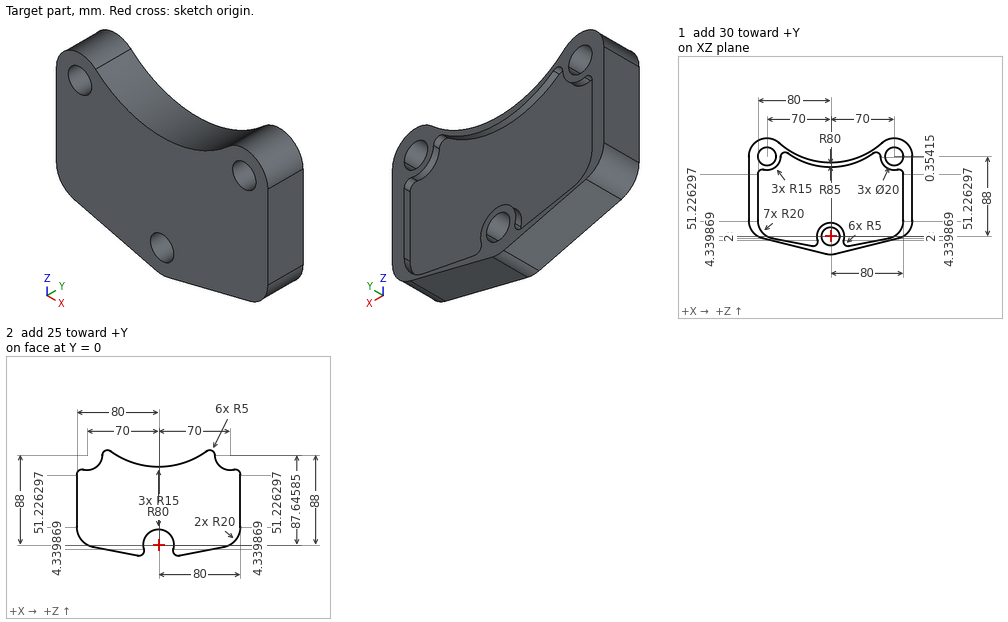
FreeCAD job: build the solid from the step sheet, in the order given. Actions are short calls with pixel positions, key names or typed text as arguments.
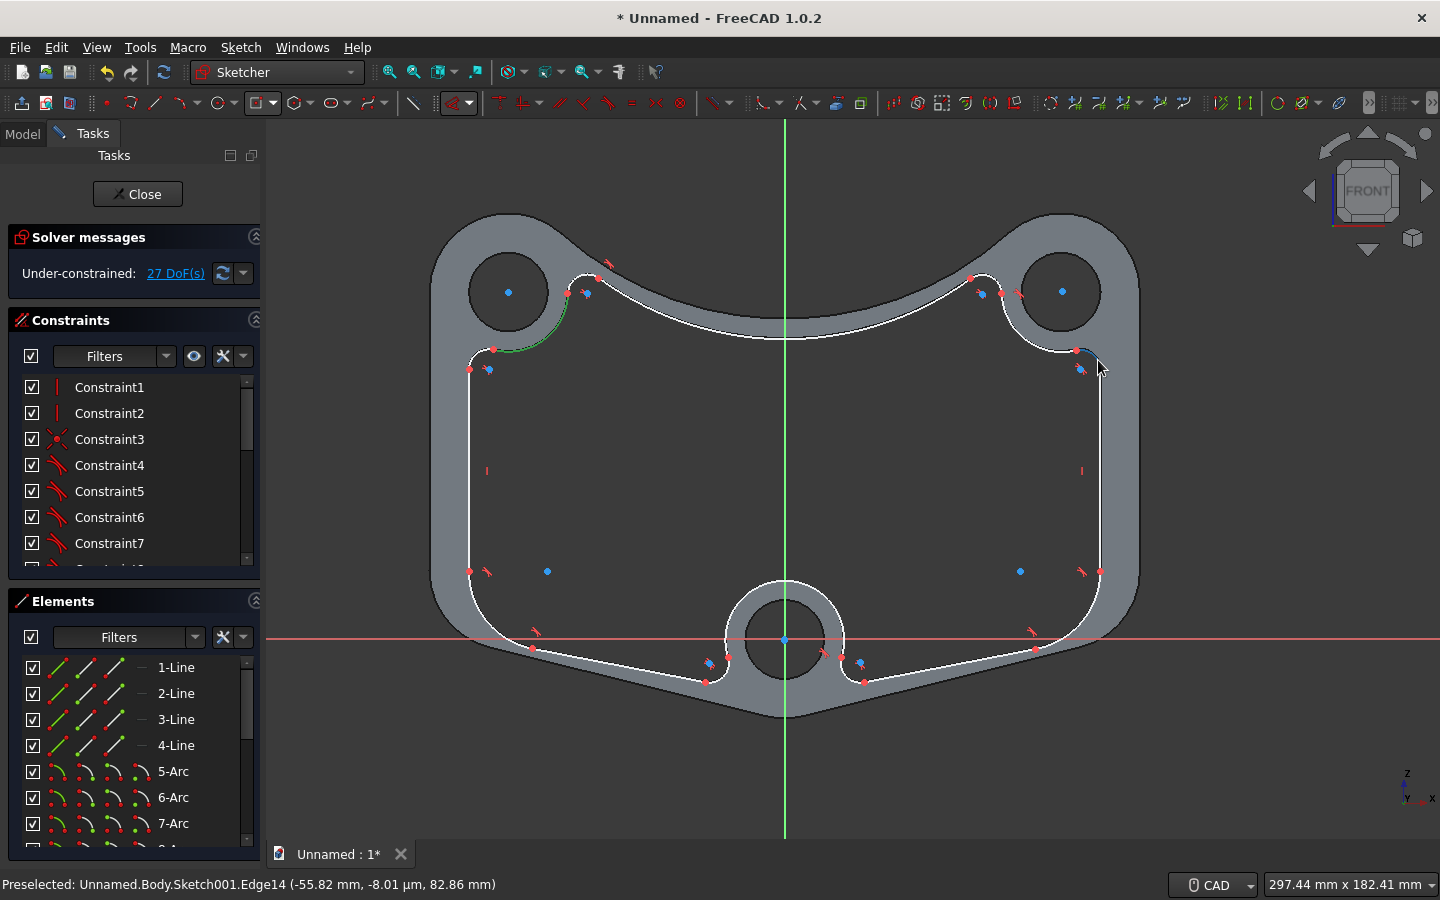
scroll(483, 350, up, 2)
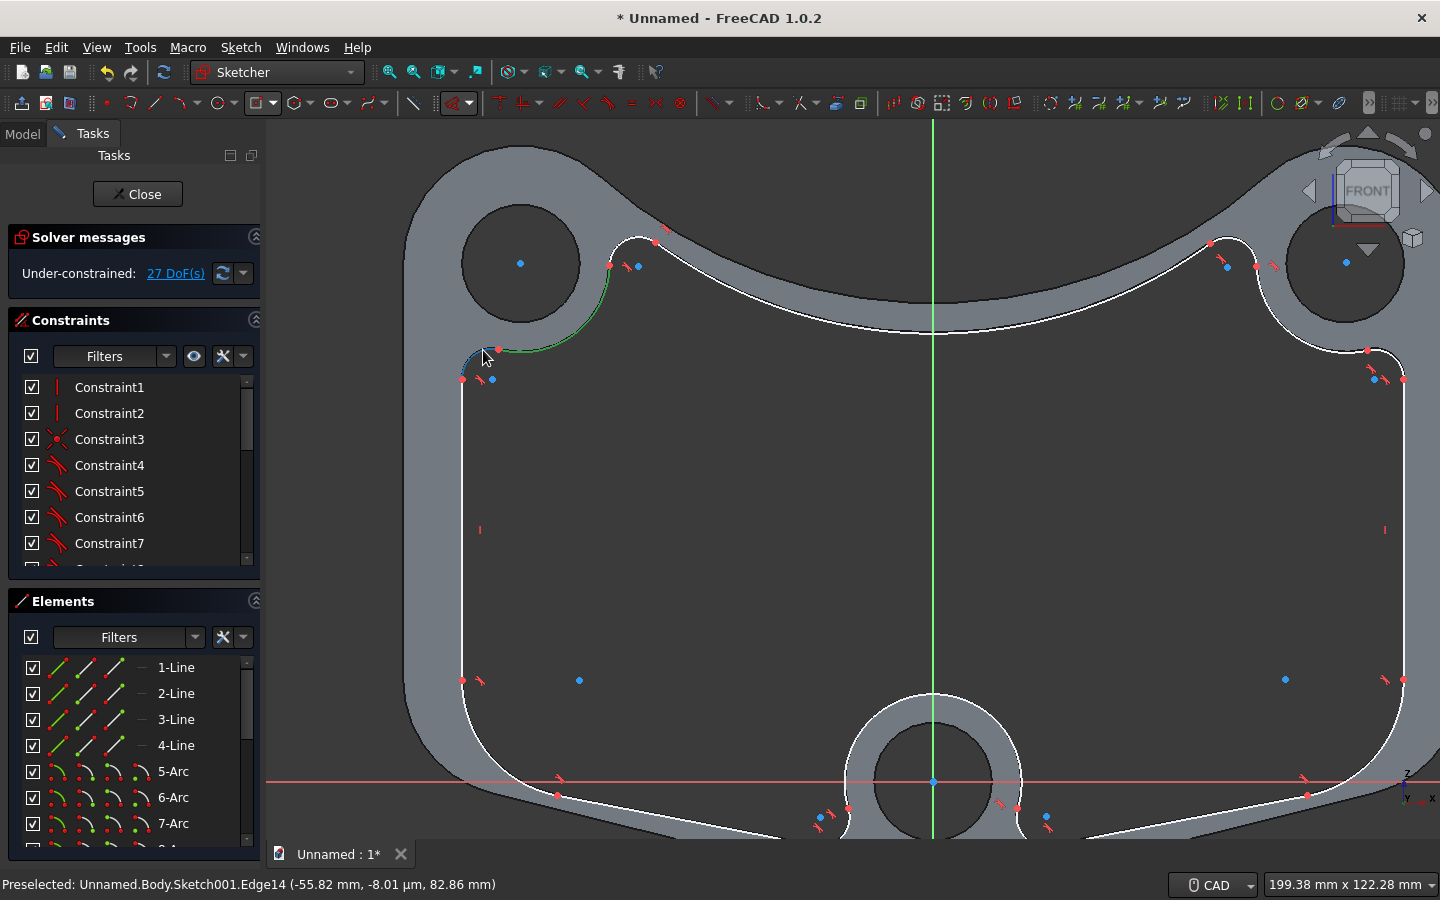
click(483, 350)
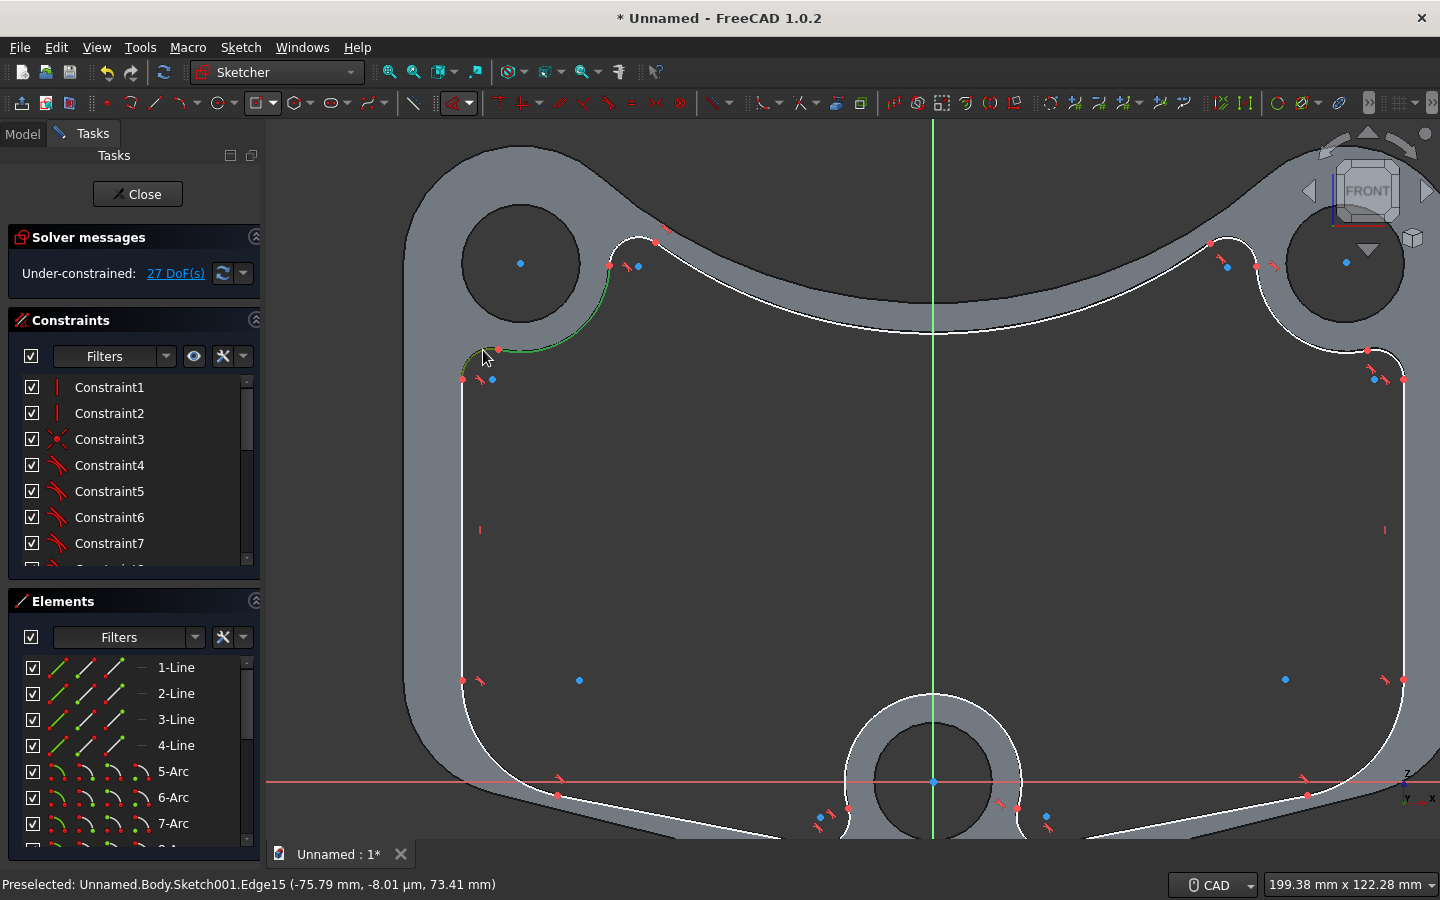
click(608, 104)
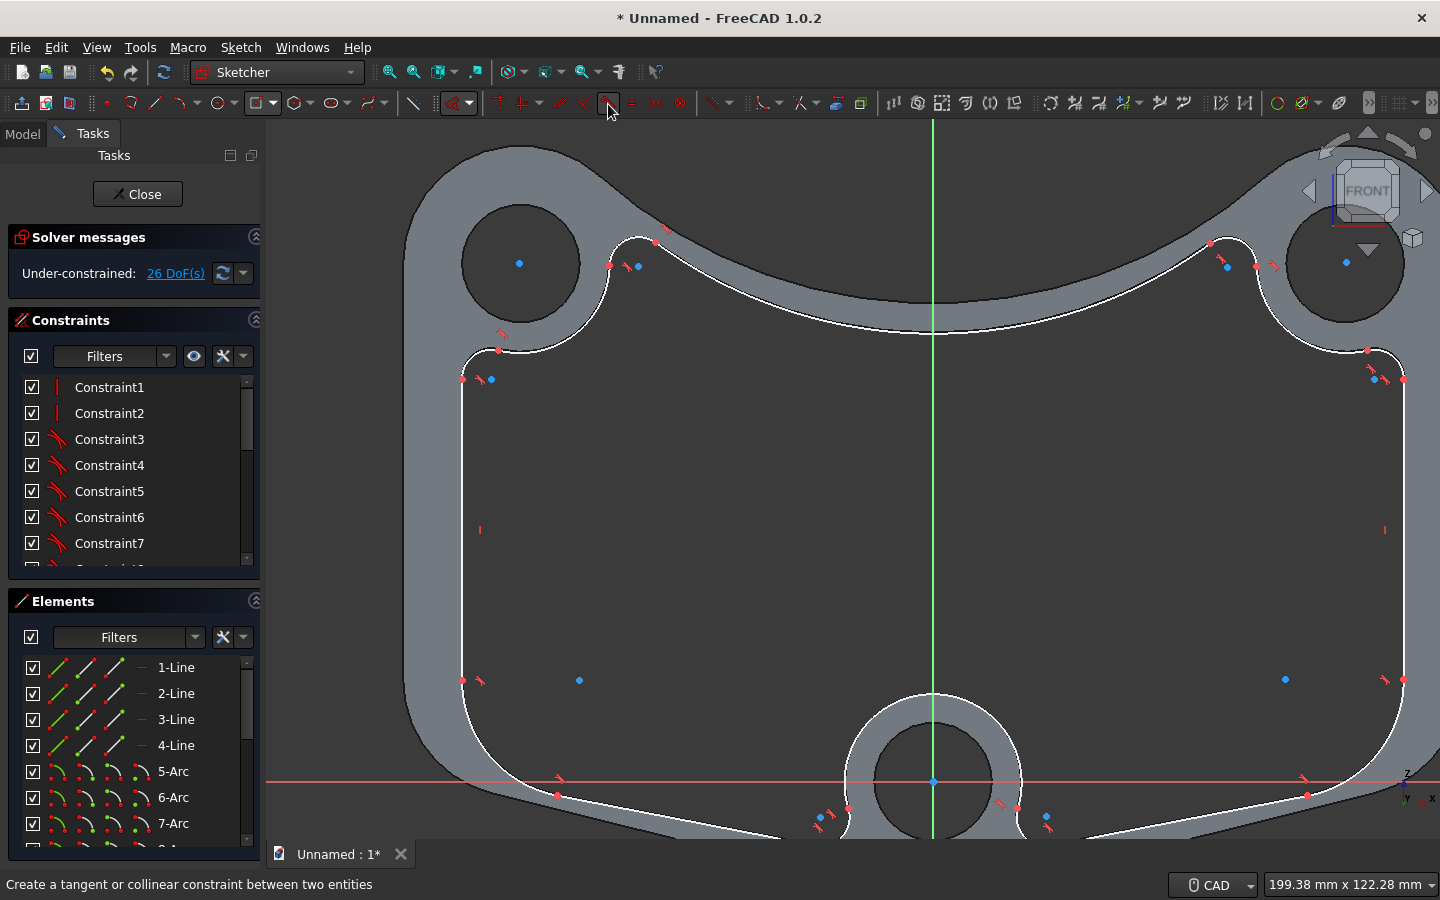
scroll(933, 782, up, 2)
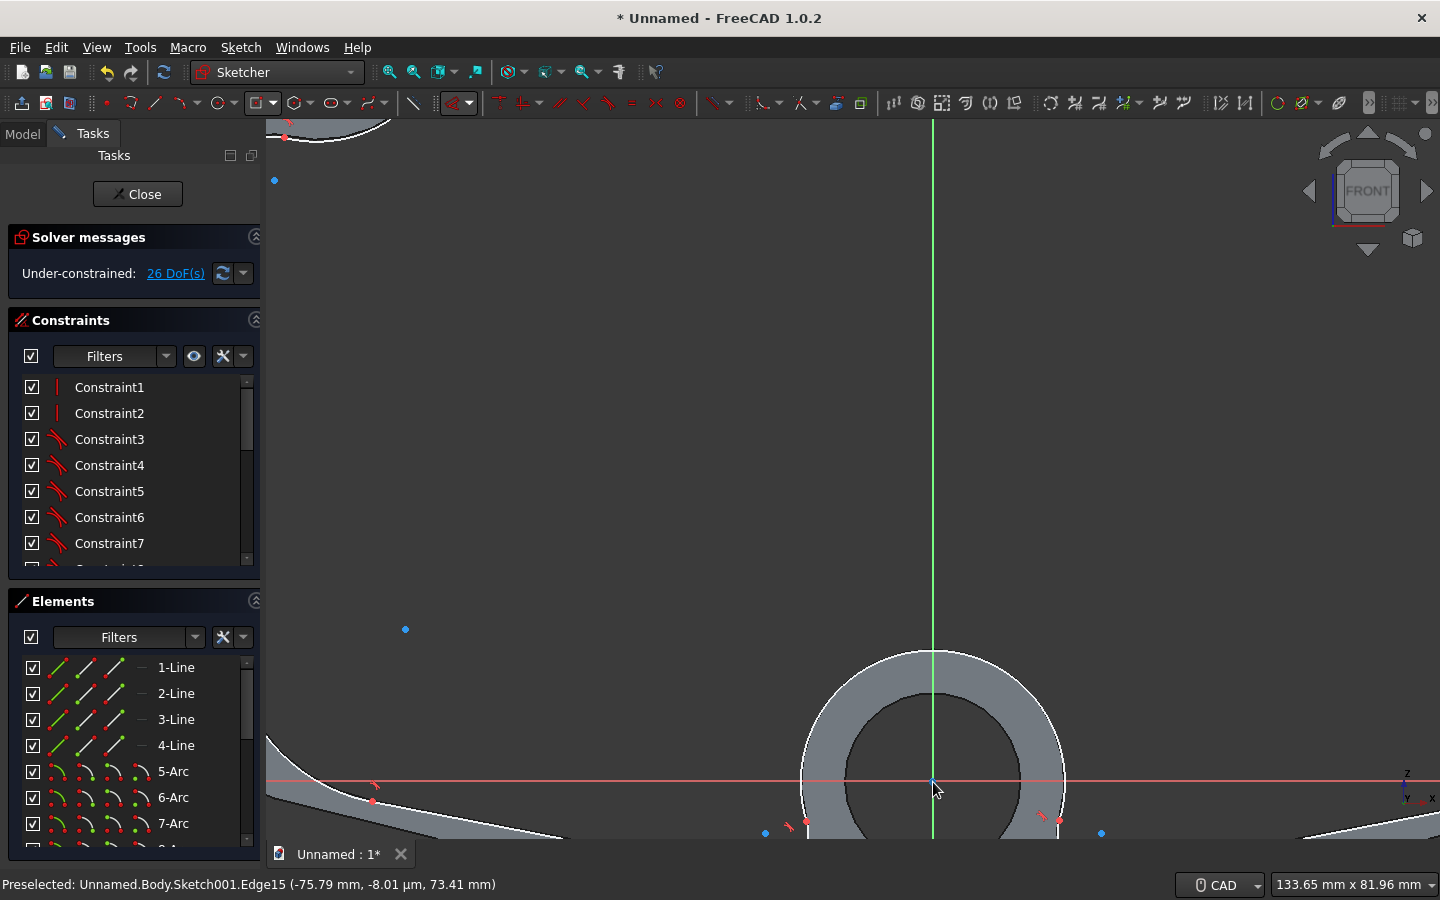
drag(923, 771, 943, 793)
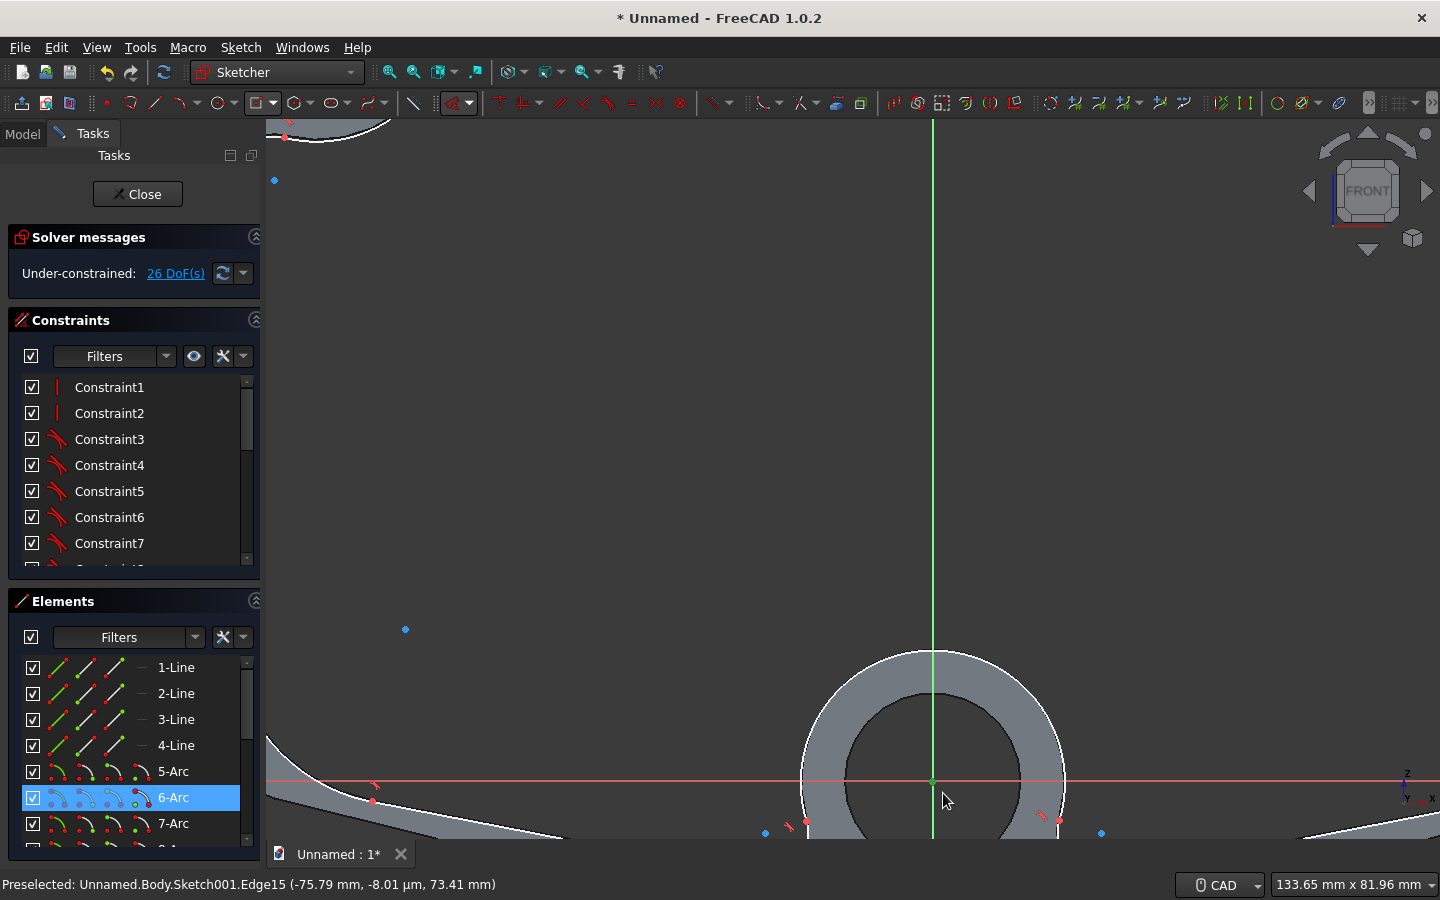
key(c)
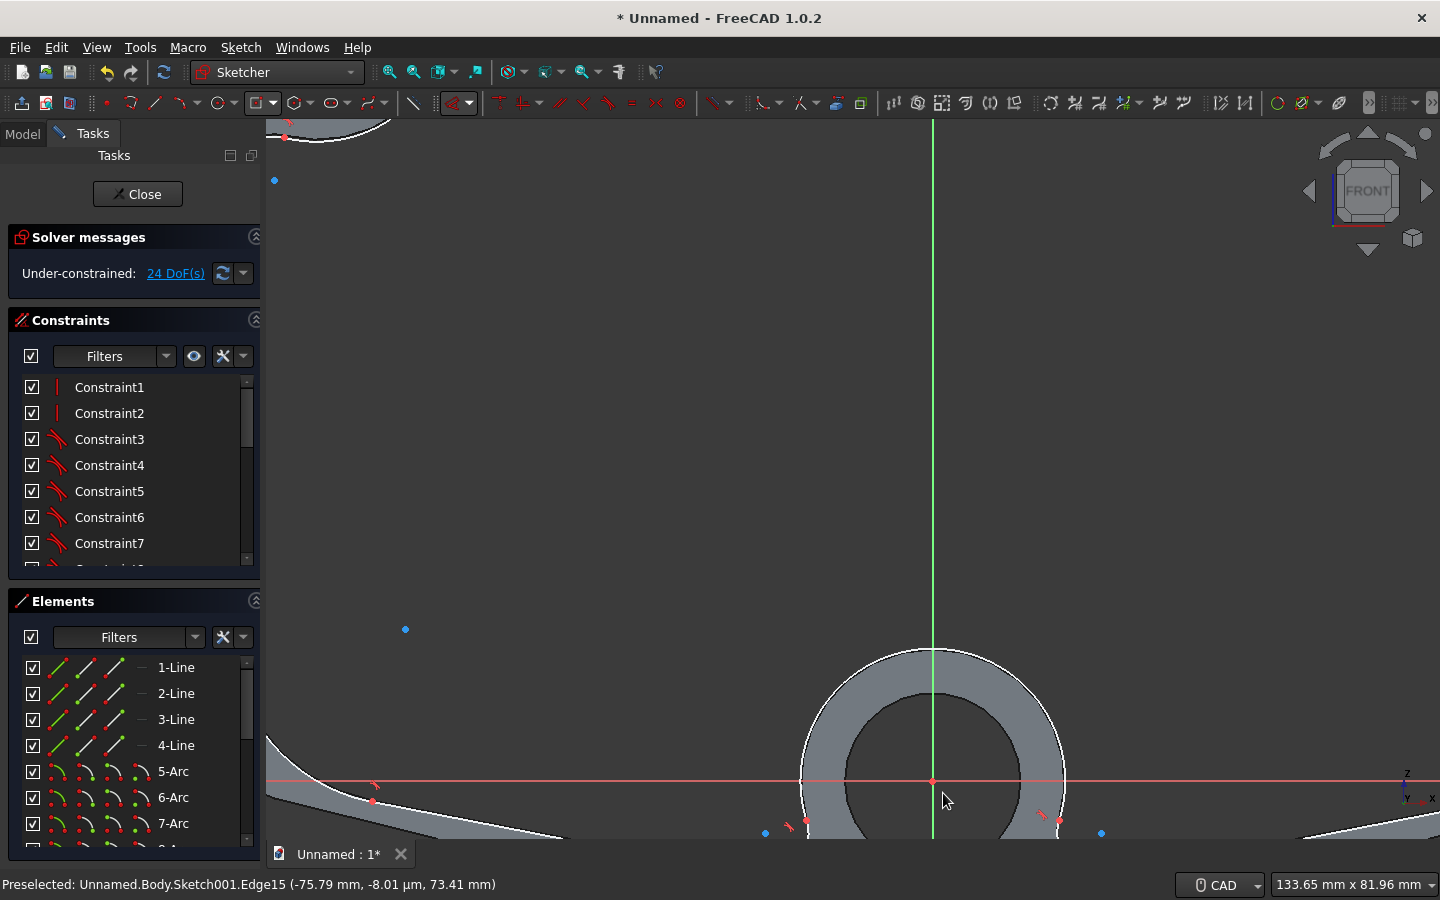
scroll(663, 524, down, 4)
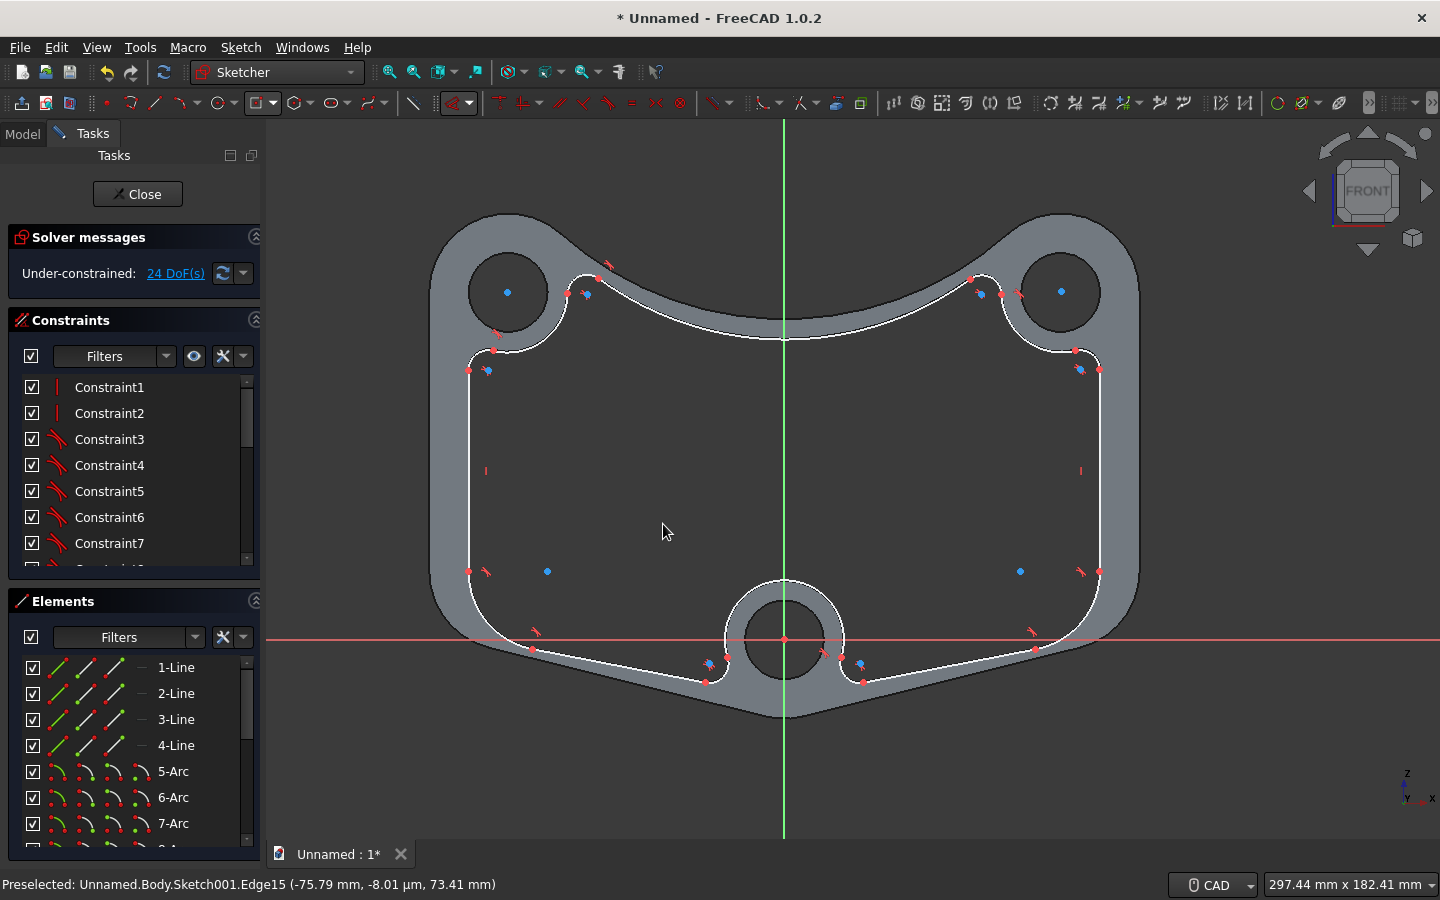
click(717, 681)